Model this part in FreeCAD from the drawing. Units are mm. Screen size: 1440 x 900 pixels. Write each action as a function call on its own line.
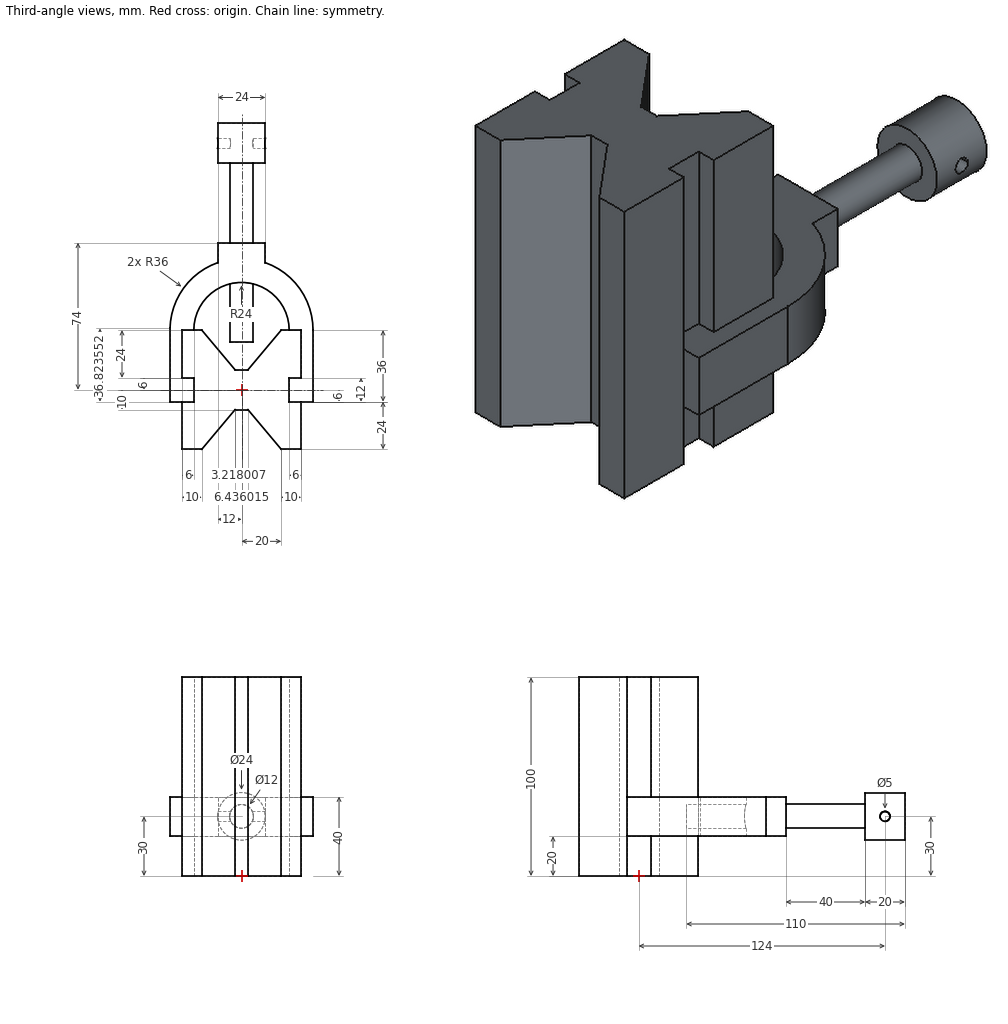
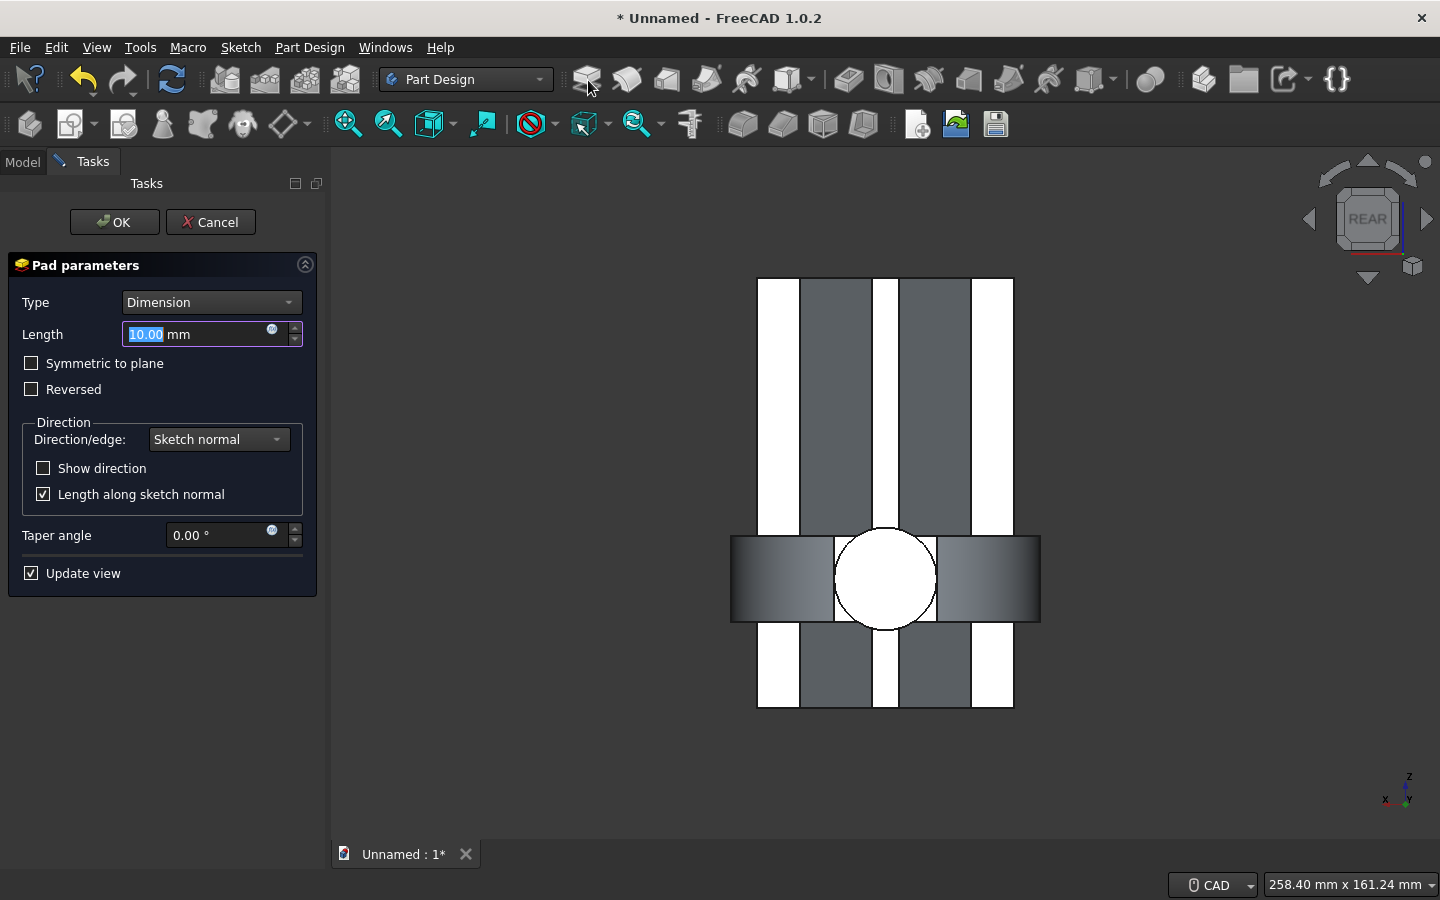
text(20)
key(Tab)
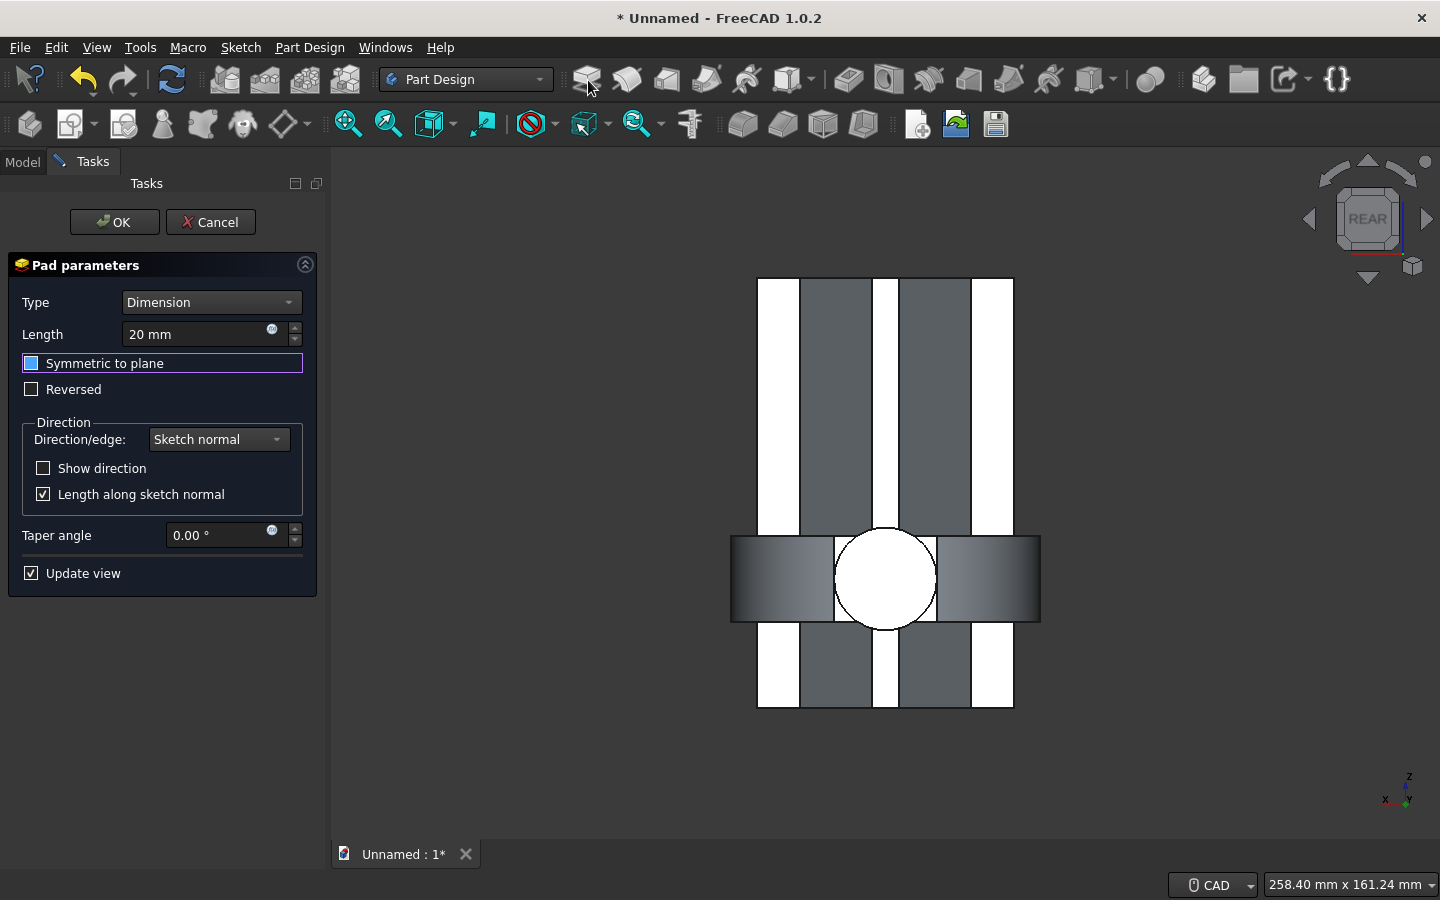
click(115, 222)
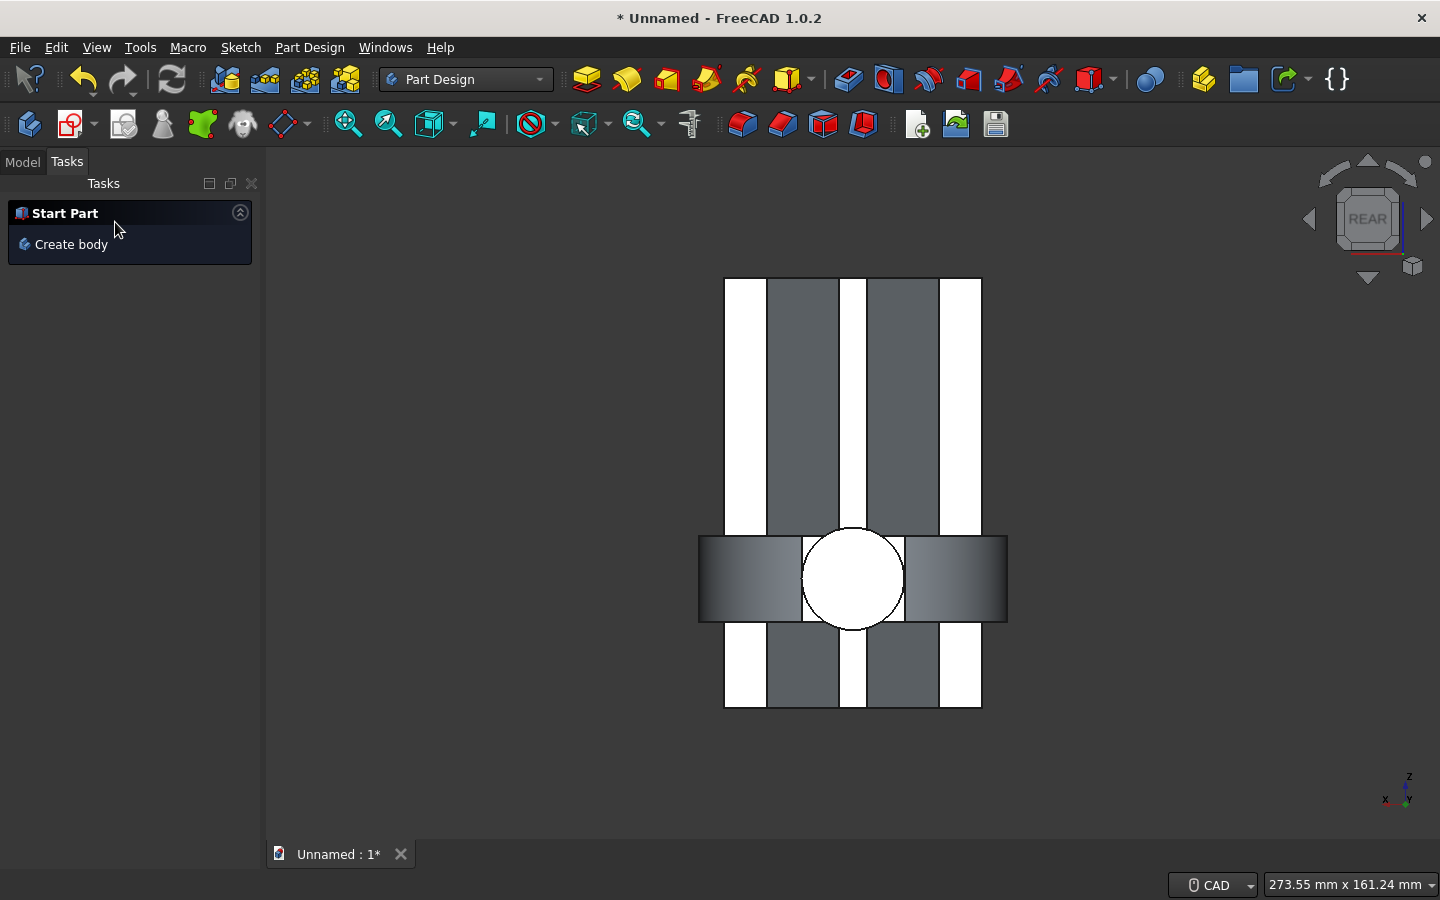
click(70, 124)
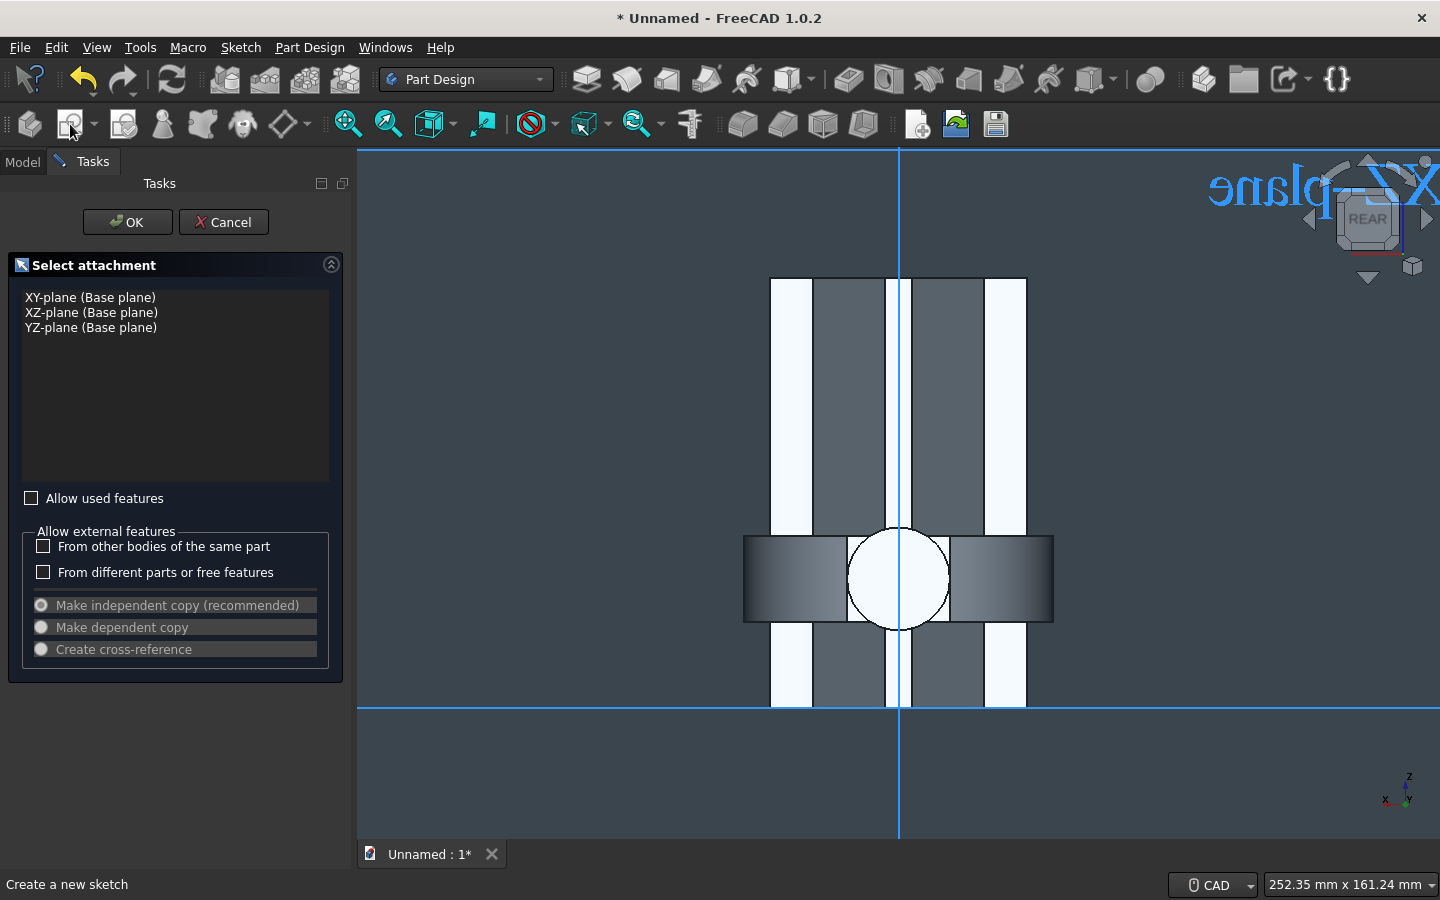
click(82, 328)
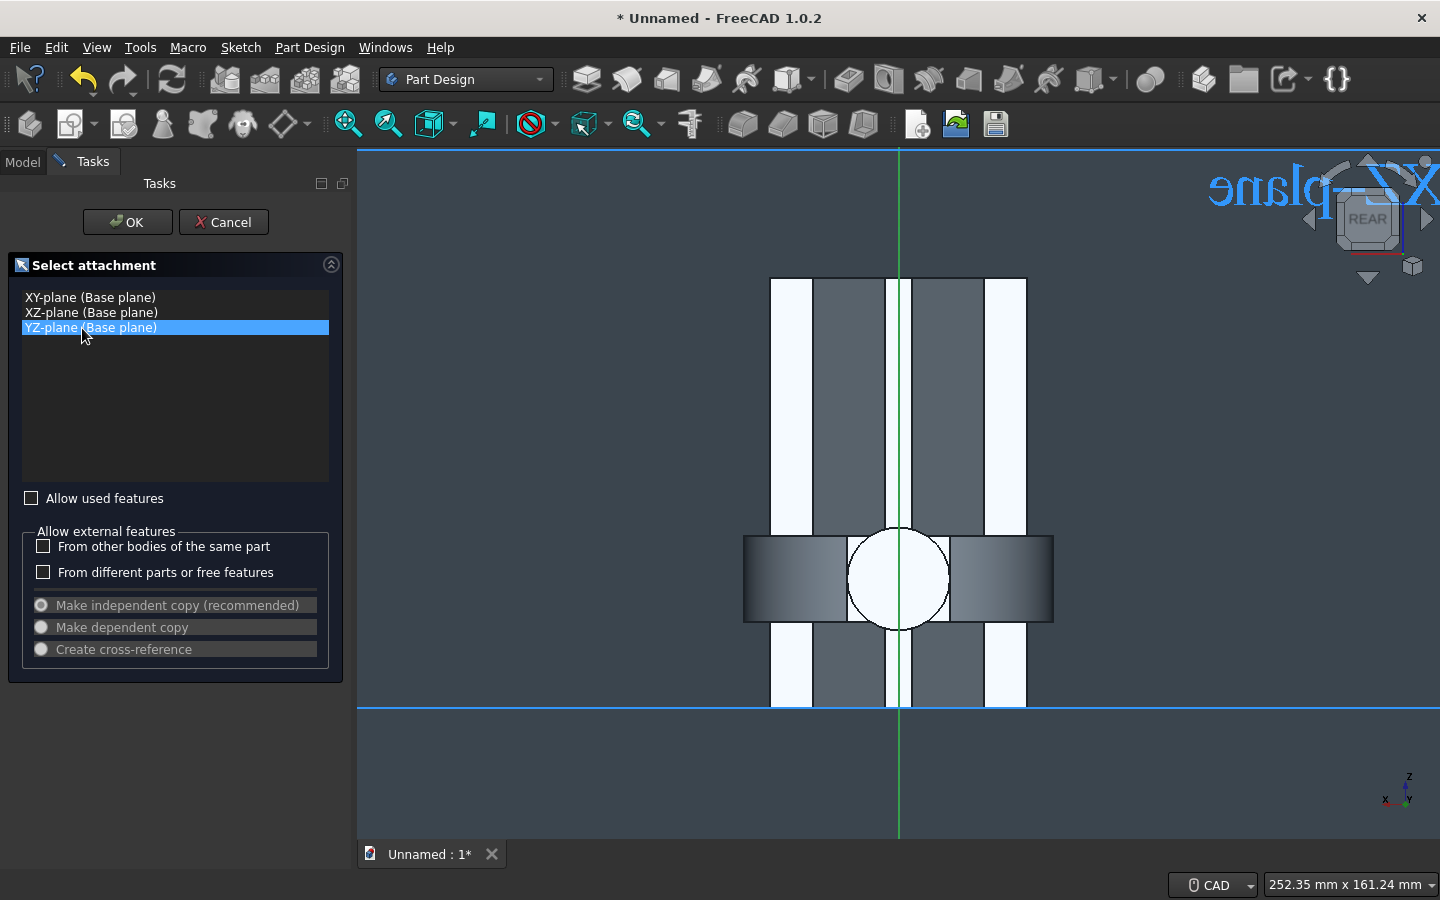
click(128, 222)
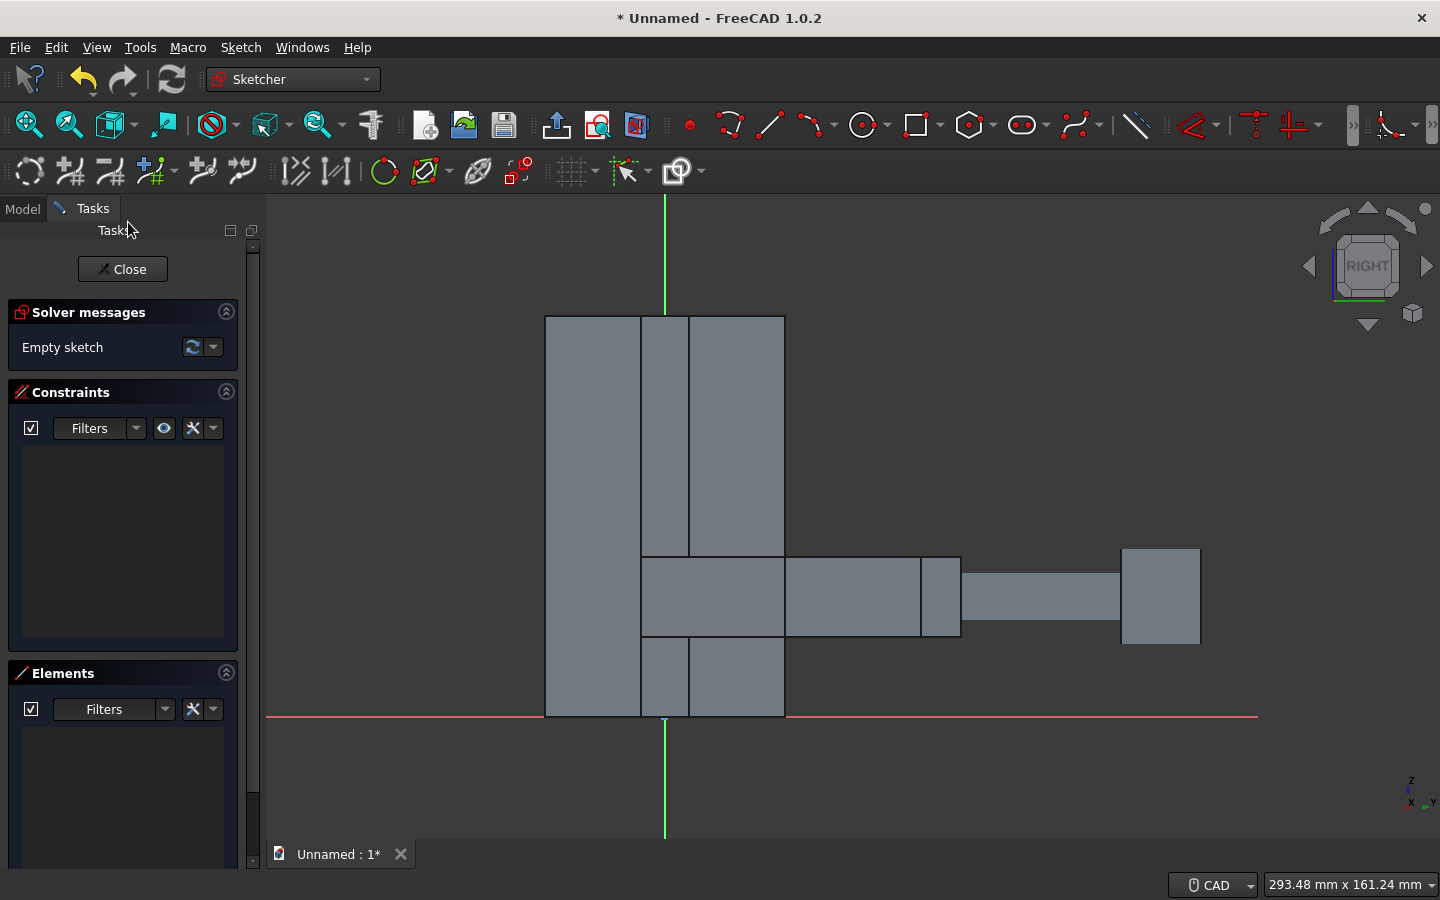
key(q)
key(s)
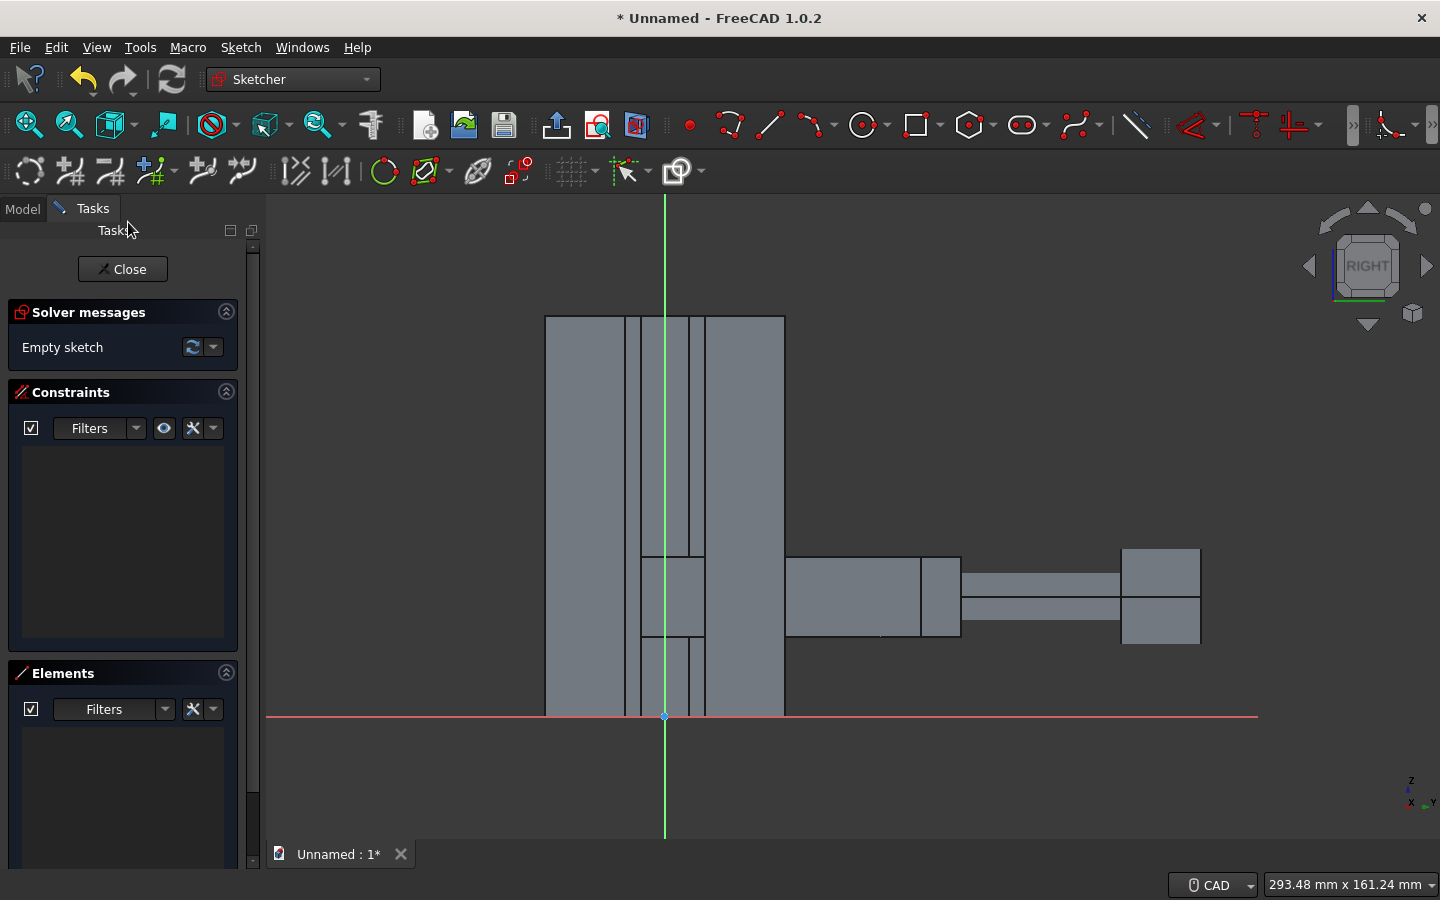
scroll(1181, 601, up, 15)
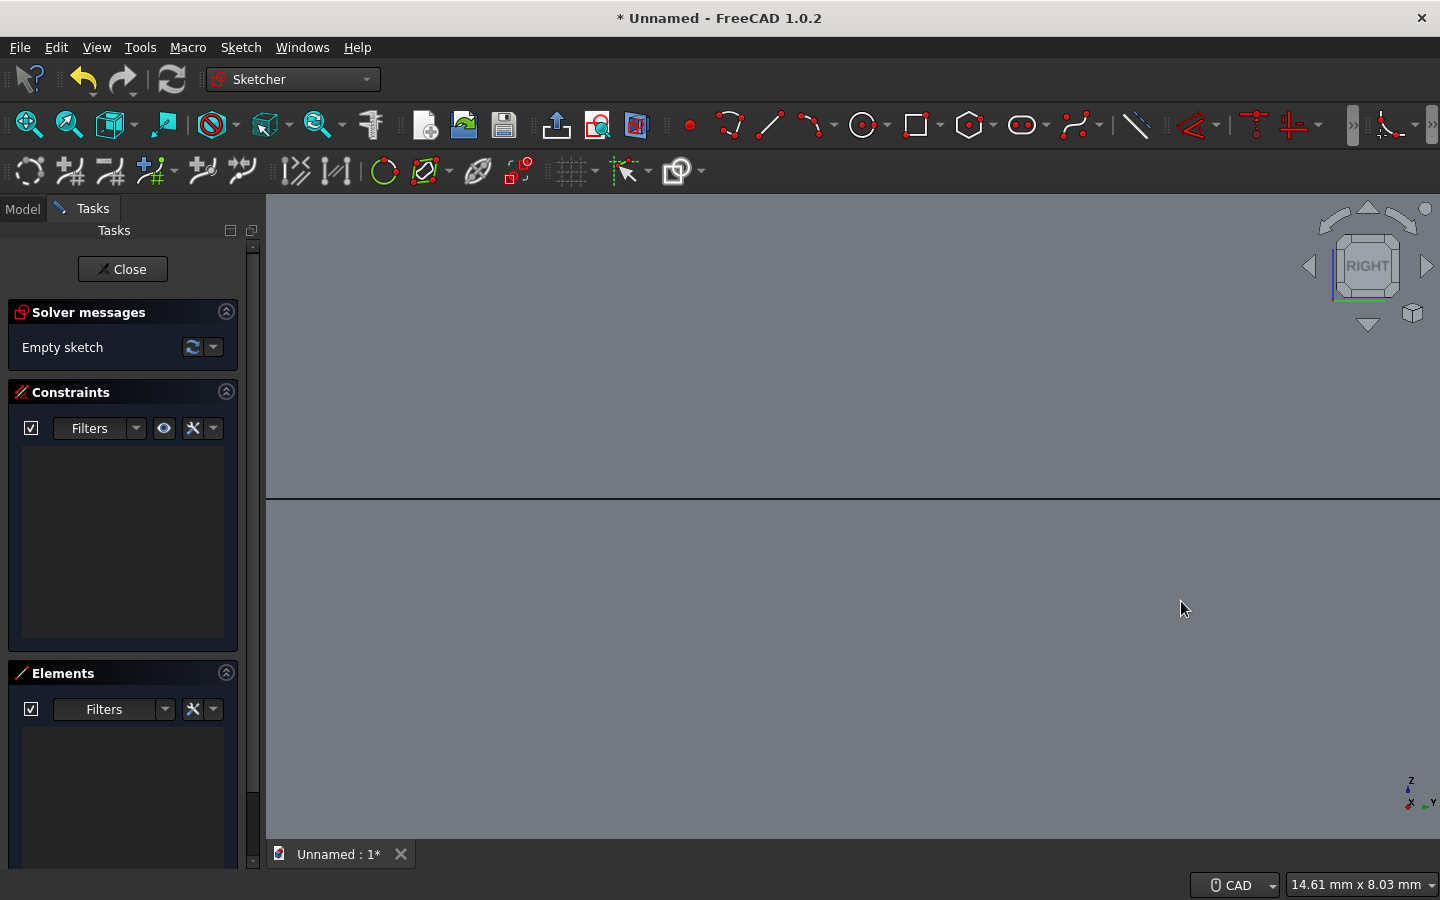
key(g)
key(c)